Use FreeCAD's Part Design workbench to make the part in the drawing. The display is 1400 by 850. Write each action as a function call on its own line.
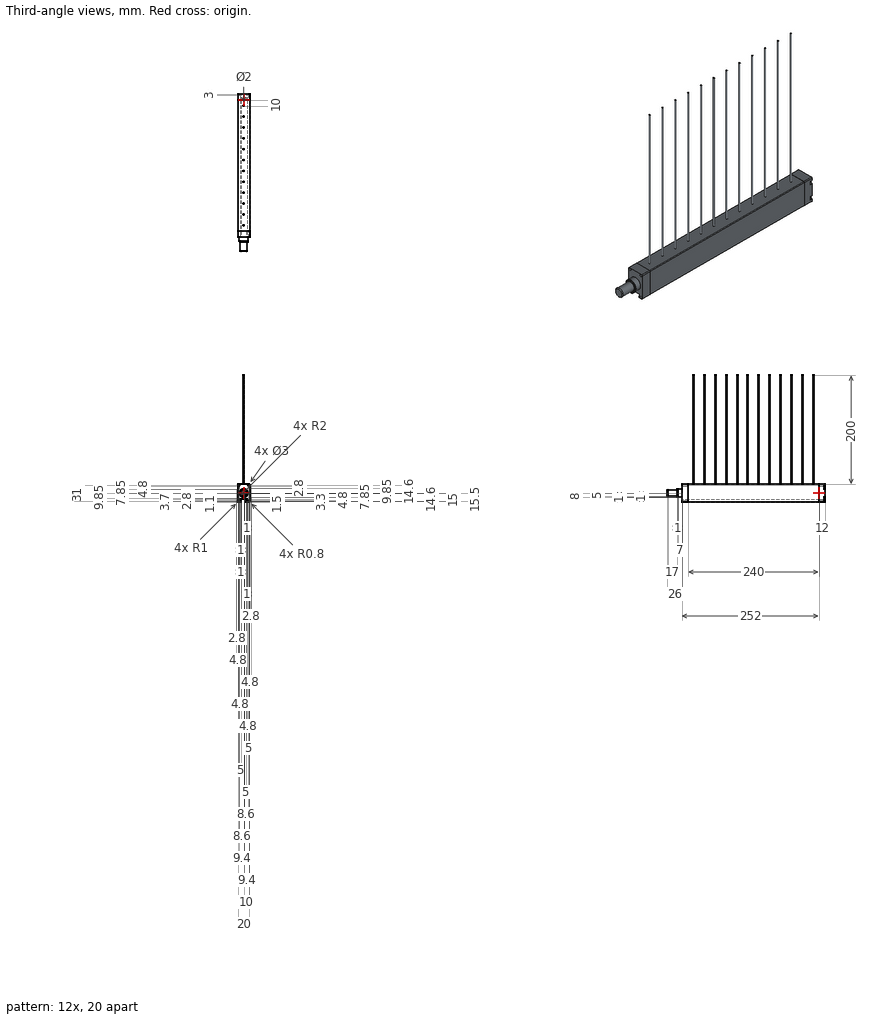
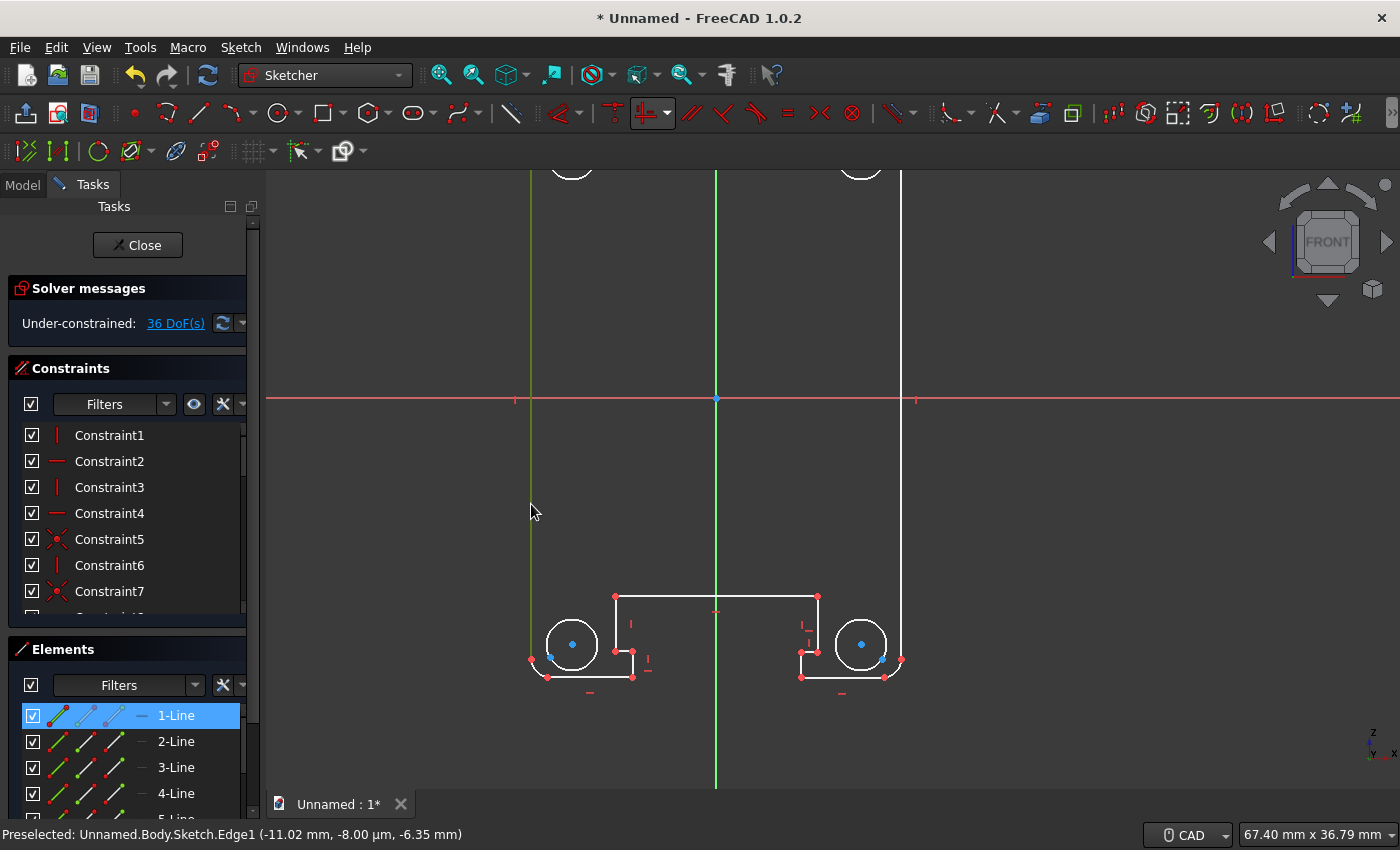
scroll(862, 645, down, 2)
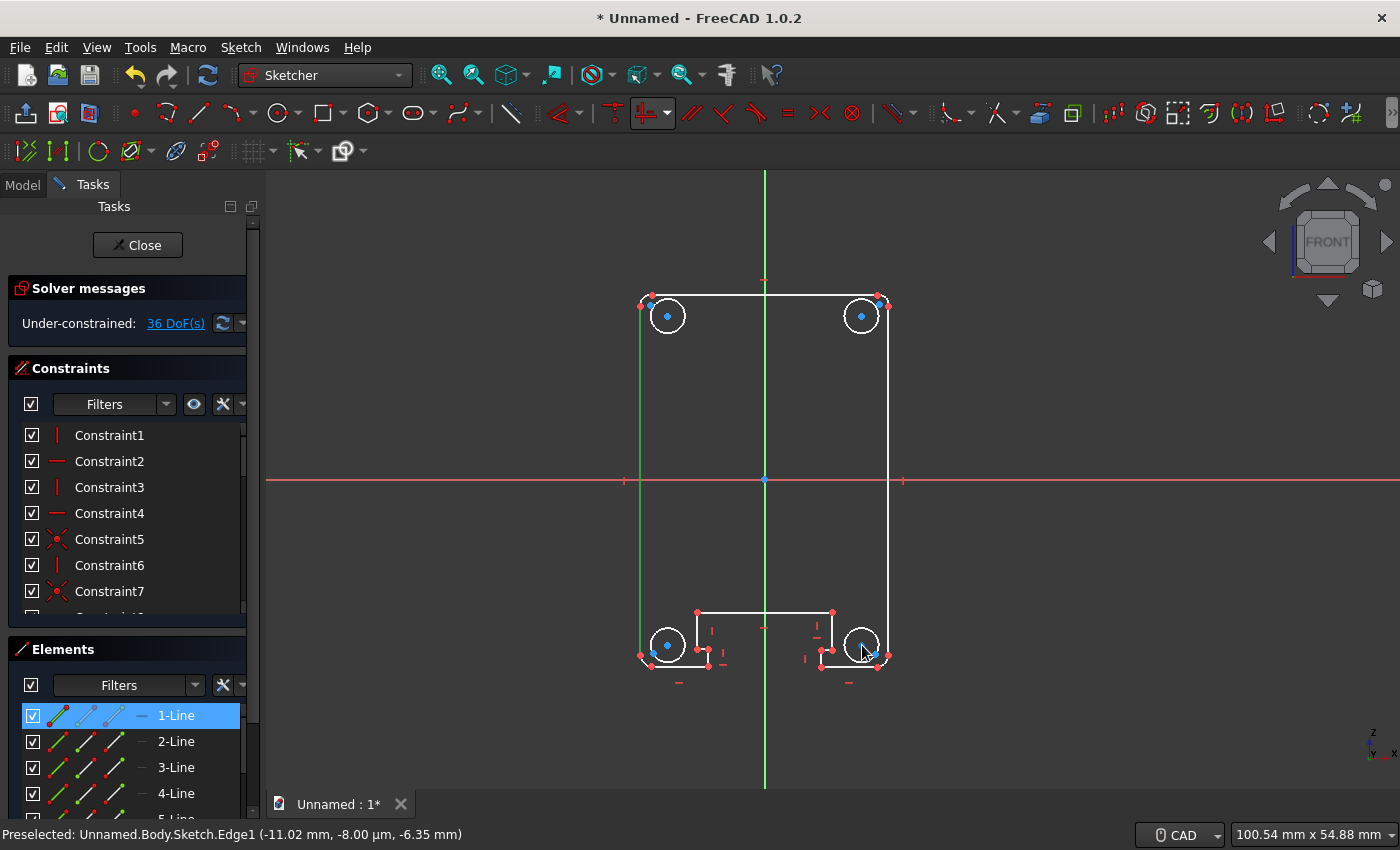
scroll(644, 298, up, 3)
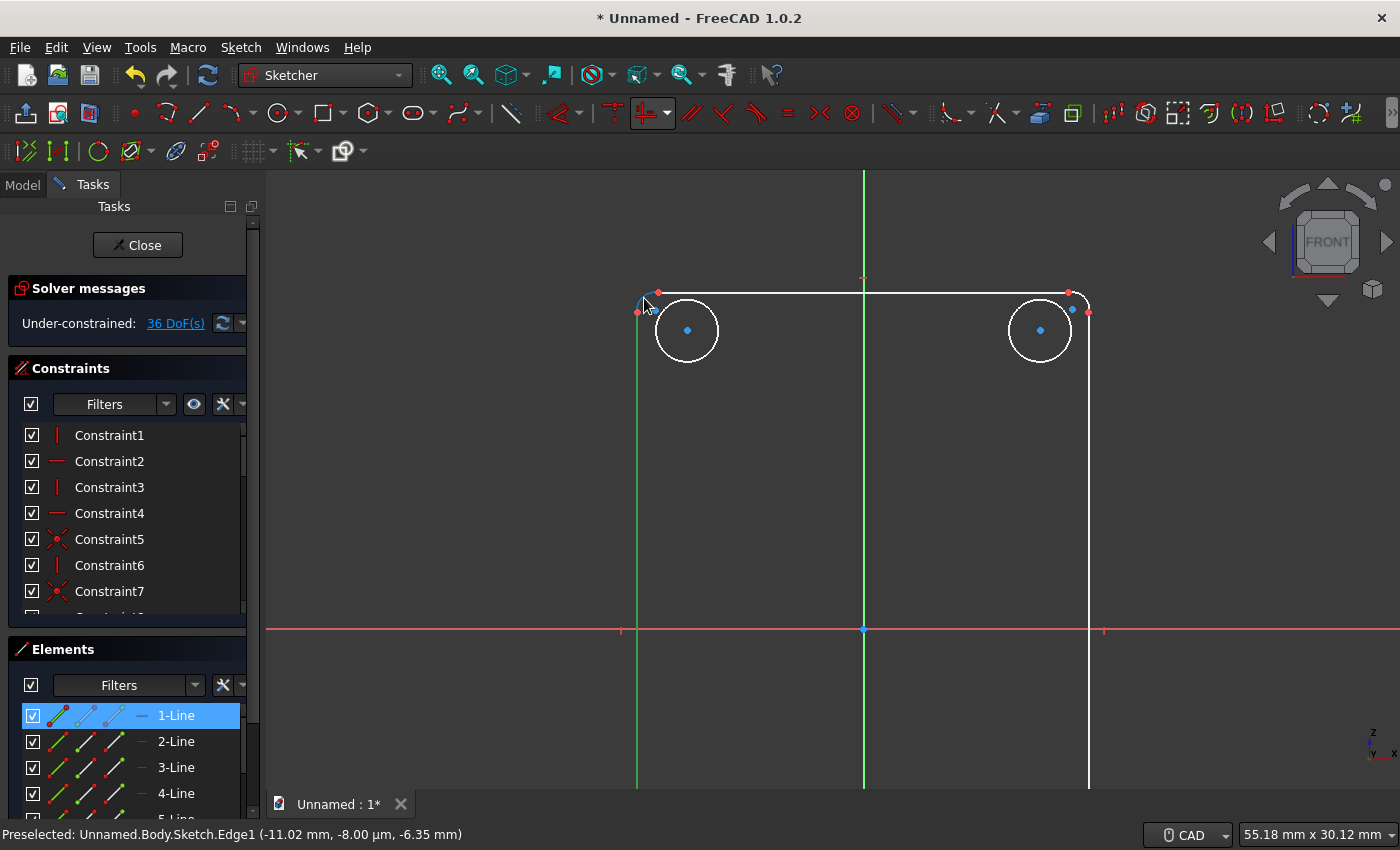
click(643, 297)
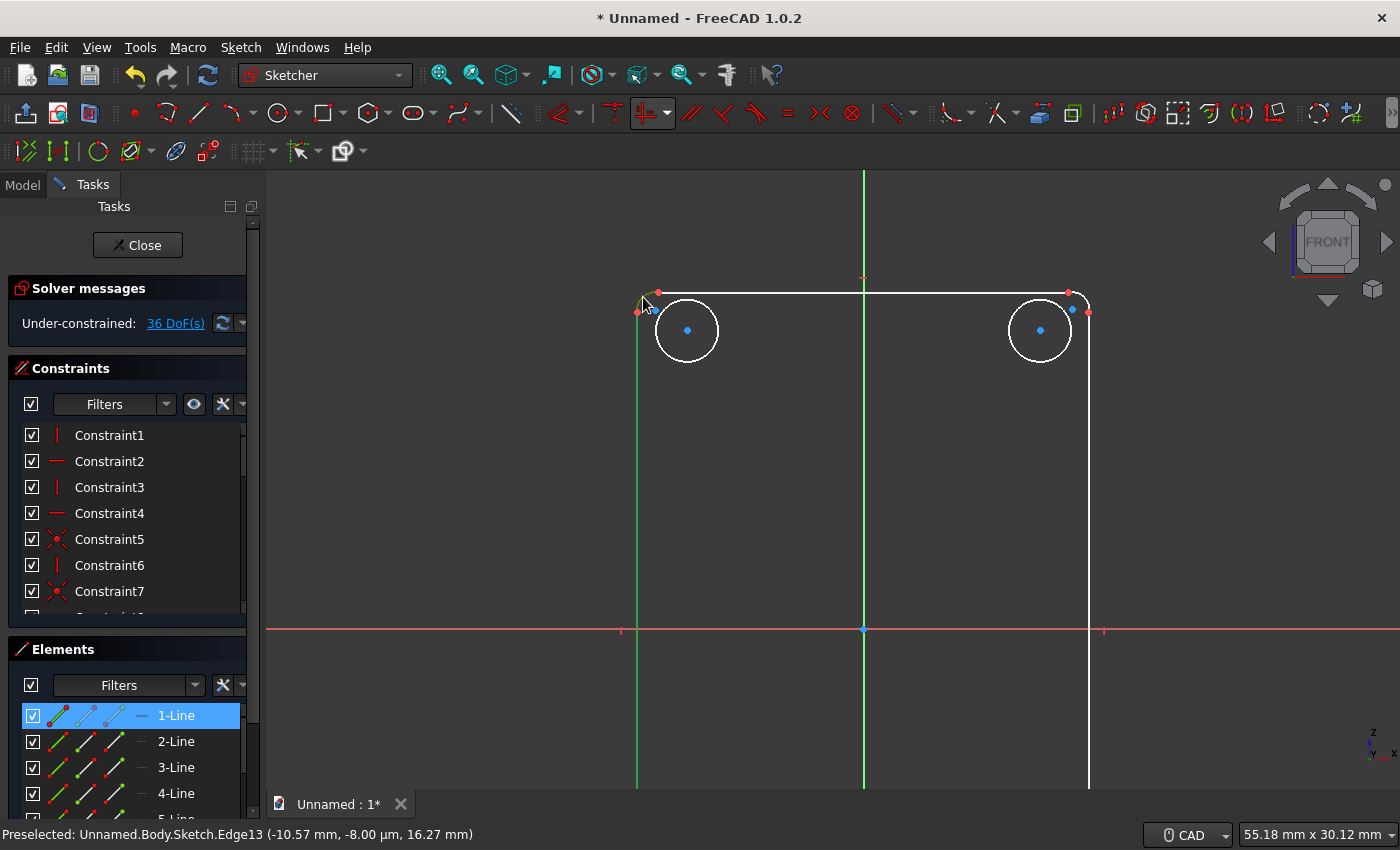
key(t)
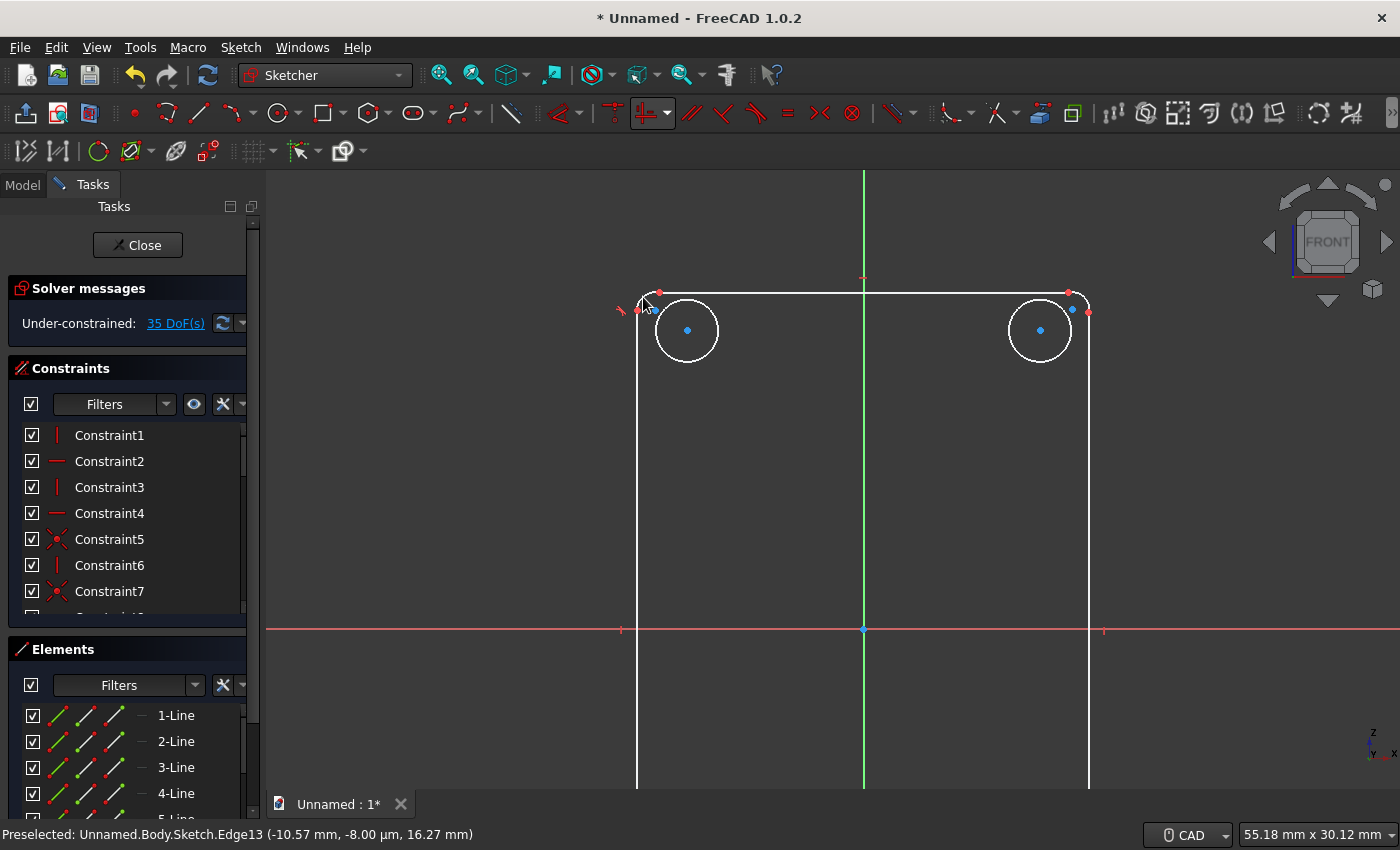
click(637, 757)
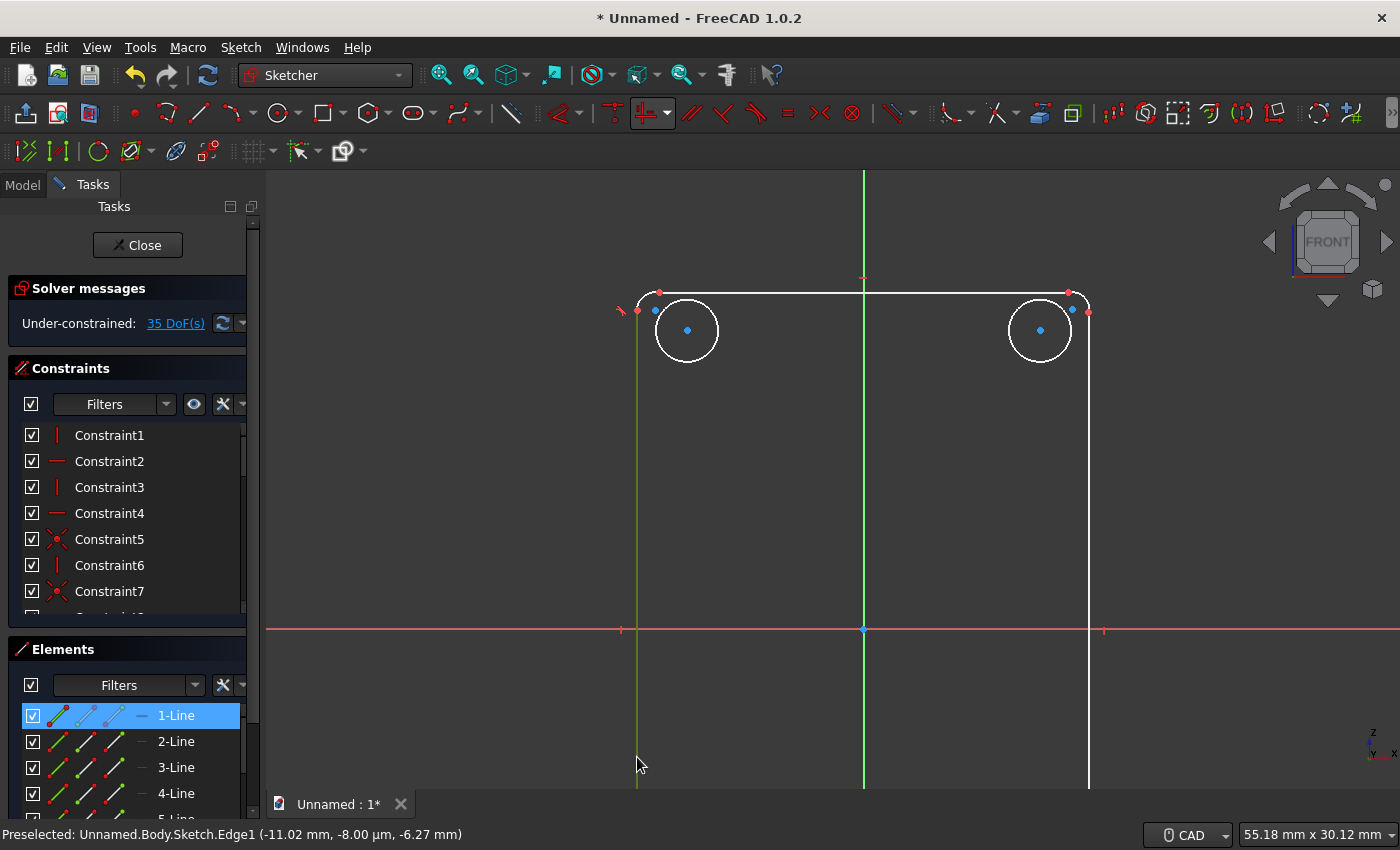
scroll(644, 298, down, 3)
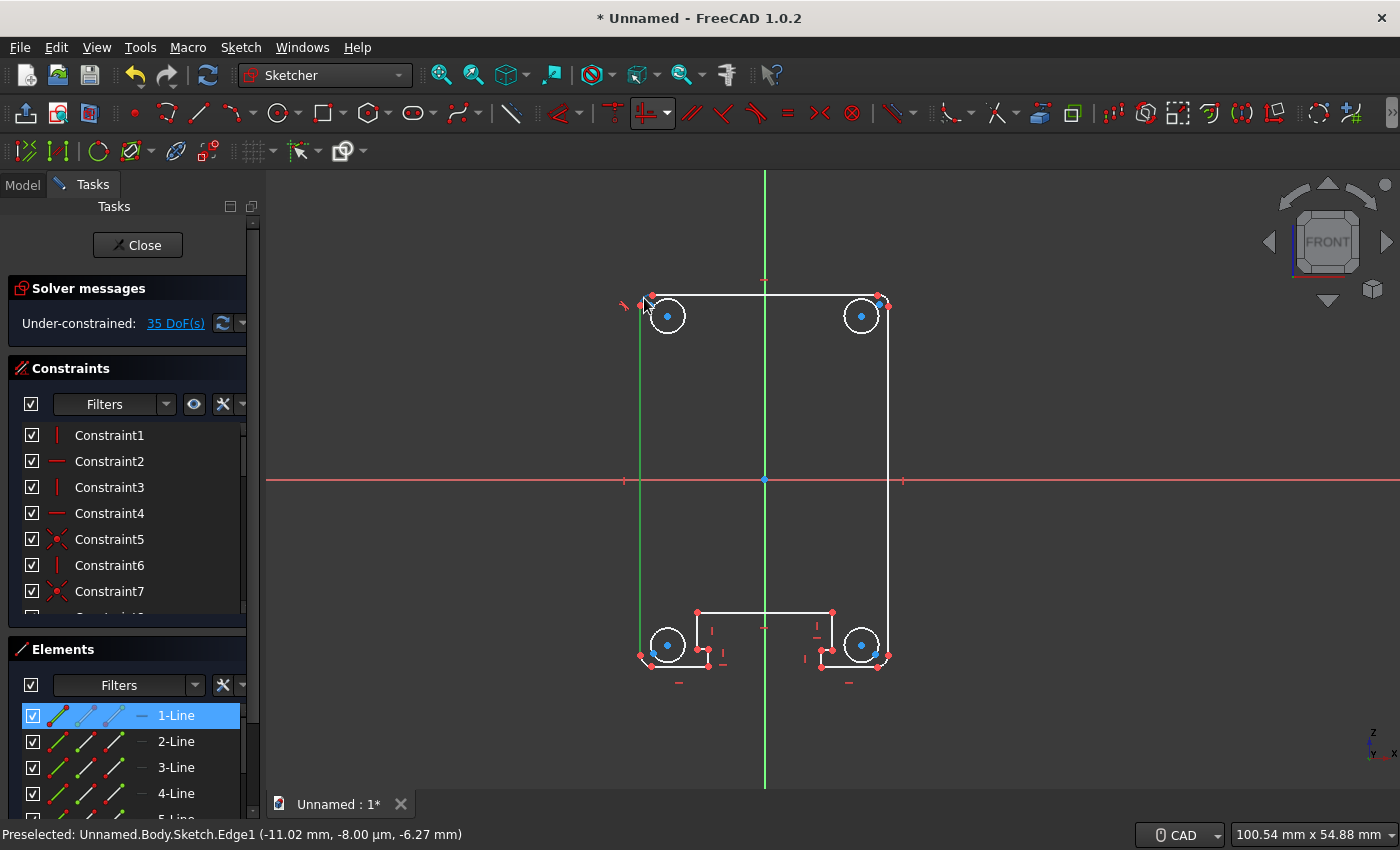
scroll(642, 660, up, 5)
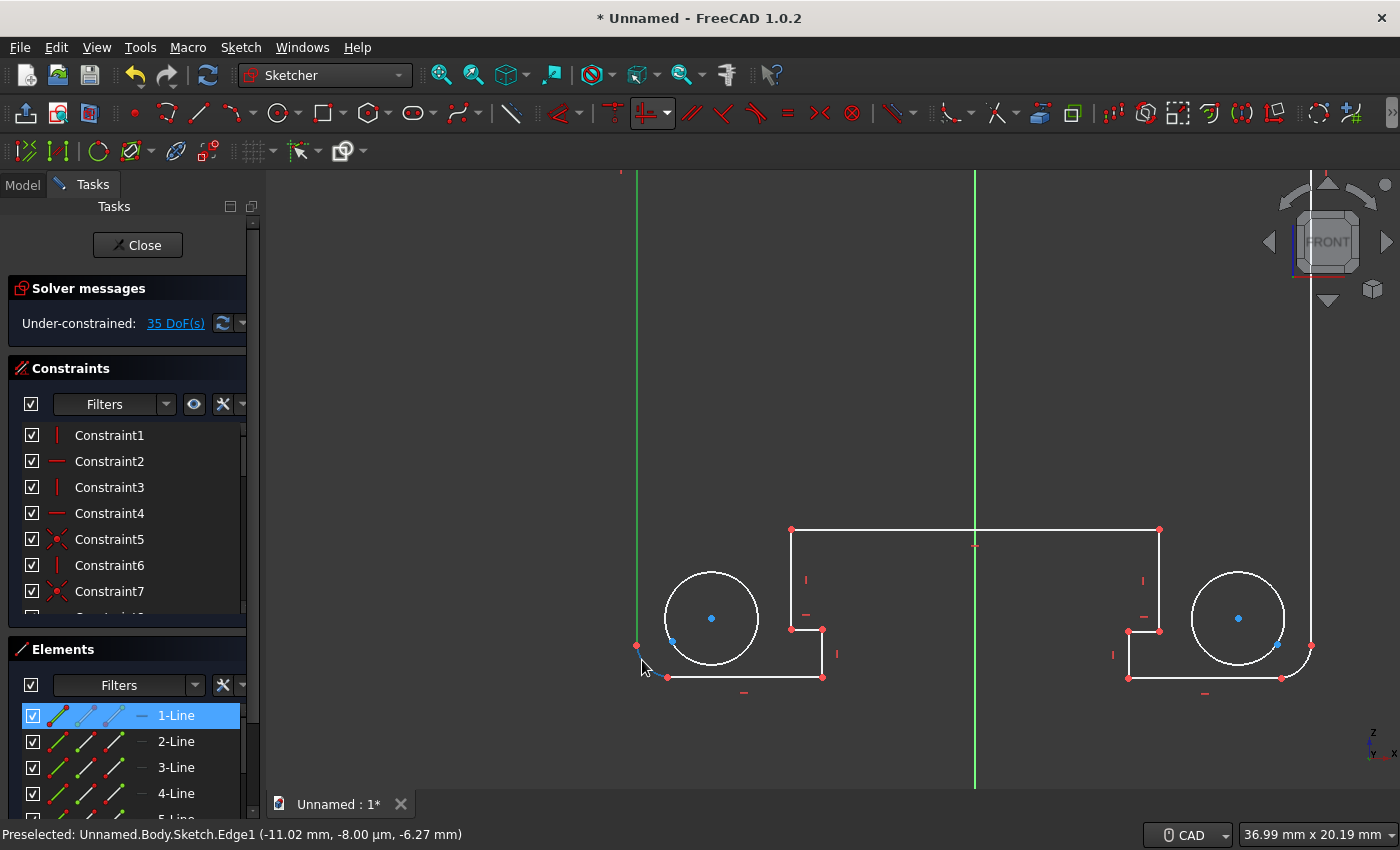
click(641, 659)